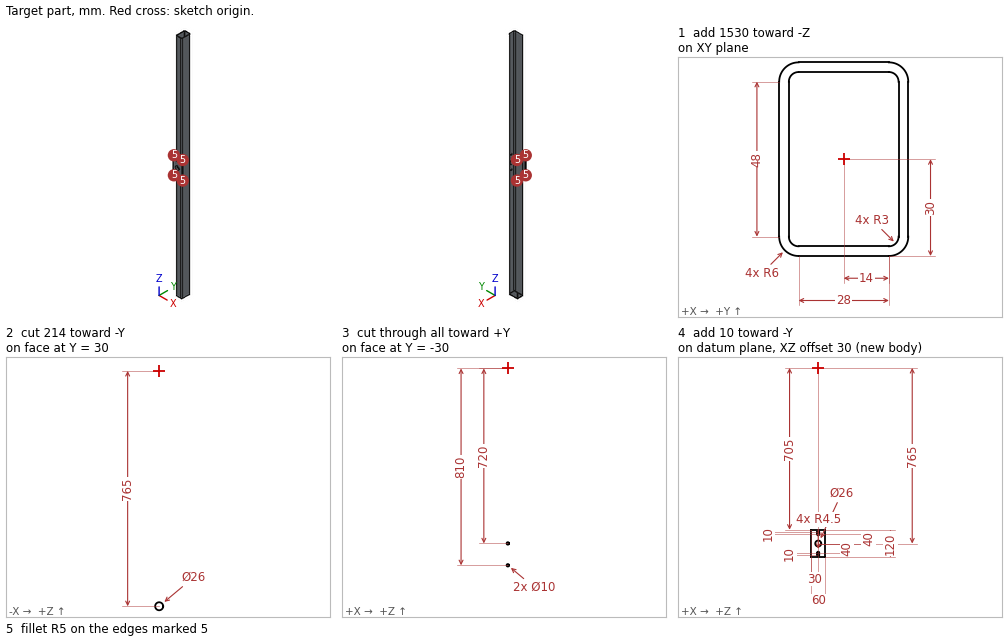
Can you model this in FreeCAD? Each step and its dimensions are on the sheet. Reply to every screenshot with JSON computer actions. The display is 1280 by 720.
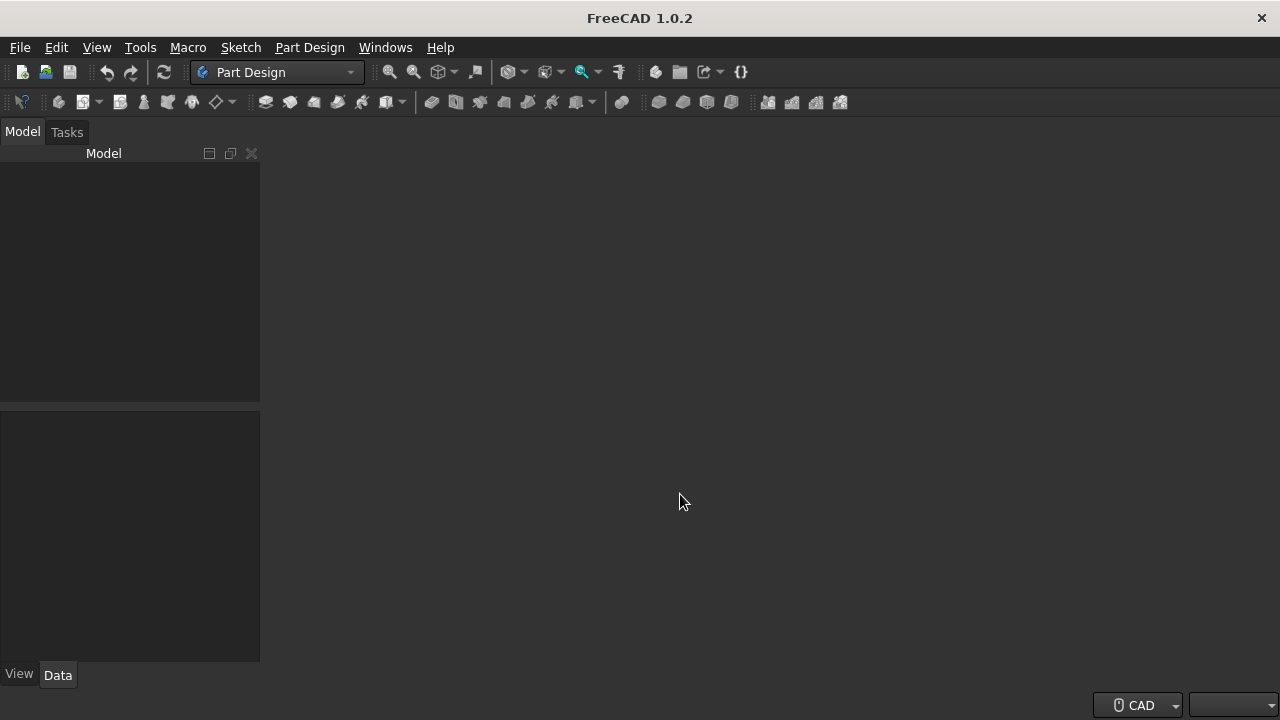
{"action": "left_click", "coordinate": [22, 72]}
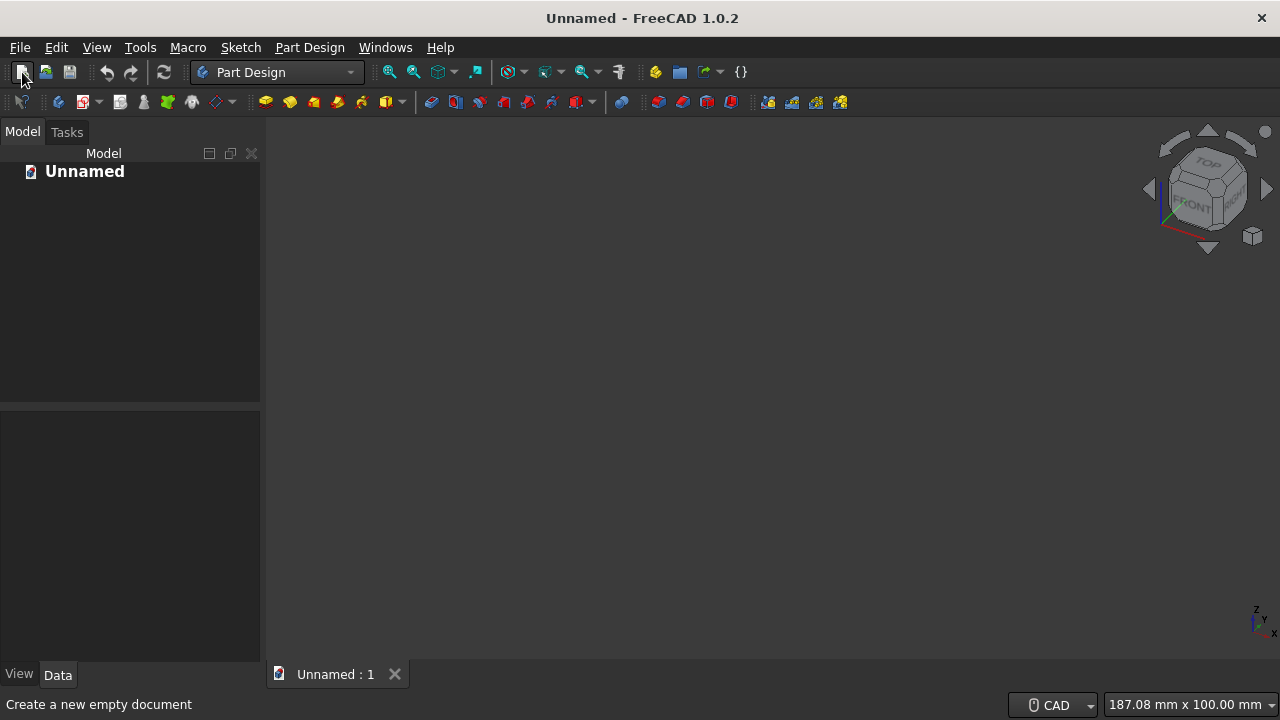
{"action": "left_click", "coordinate": [84, 102]}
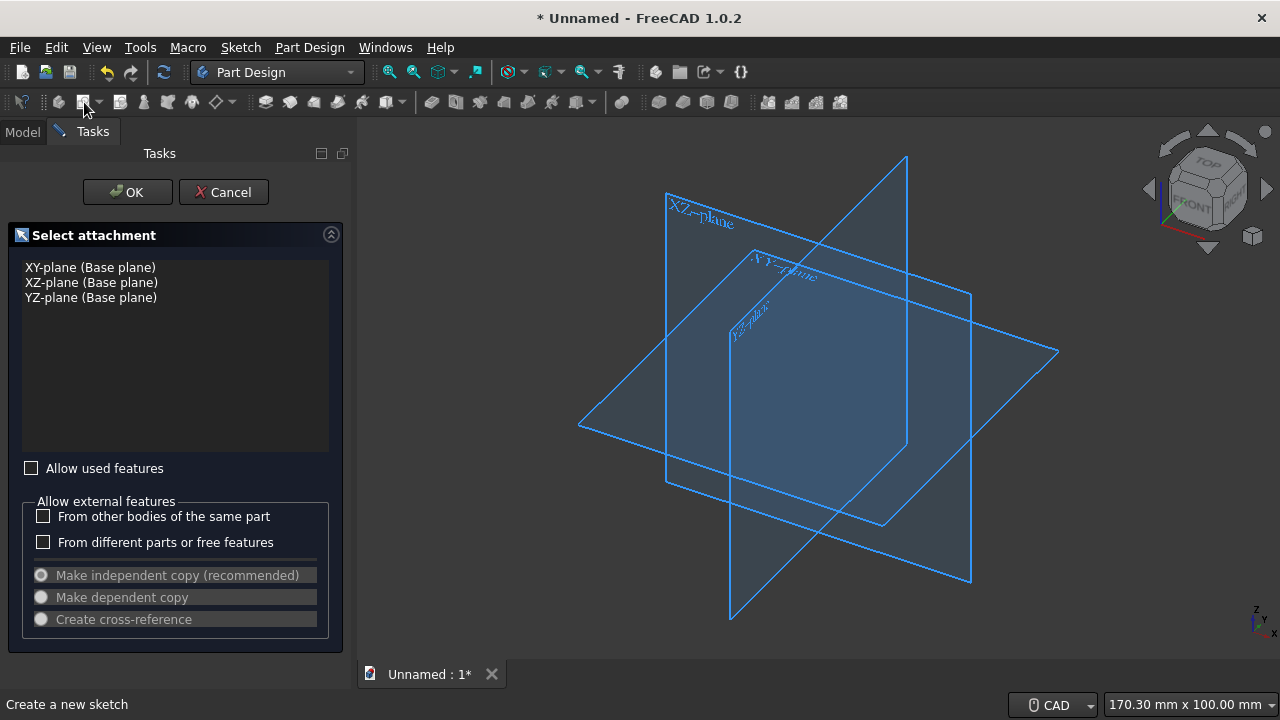
{"action": "left_click", "coordinate": [82, 268]}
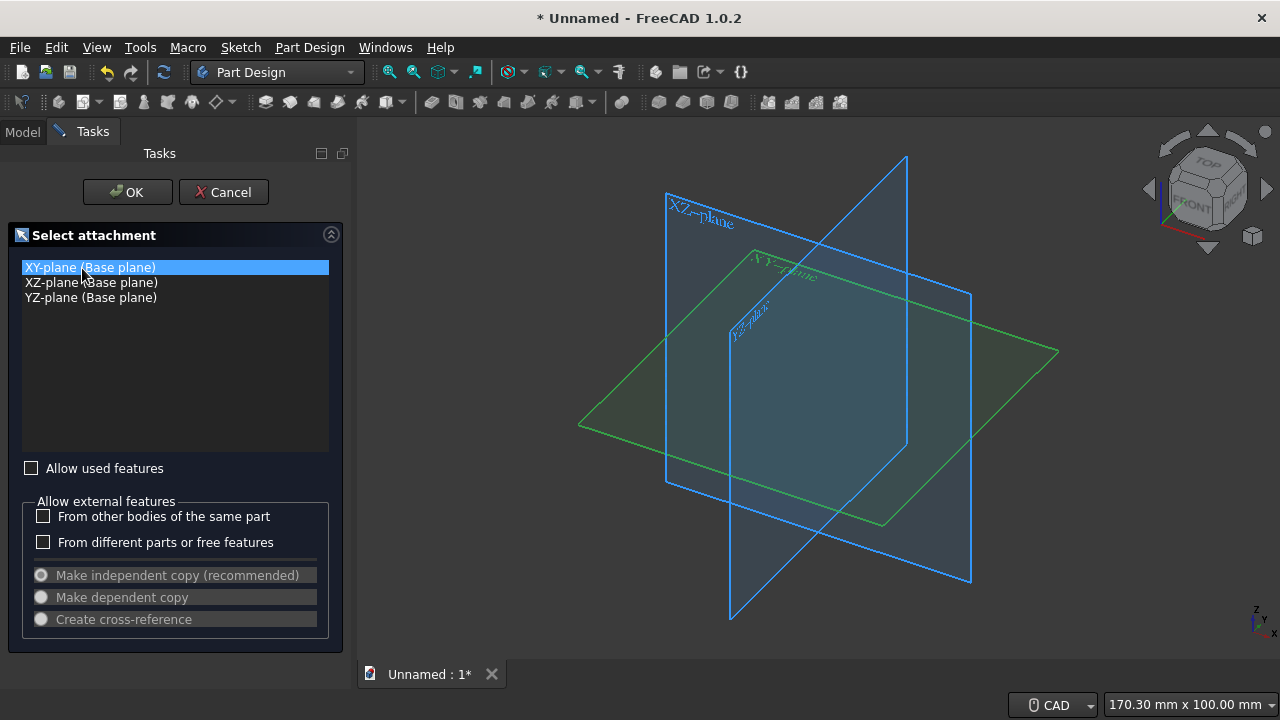
{"action": "left_click", "coordinate": [128, 192]}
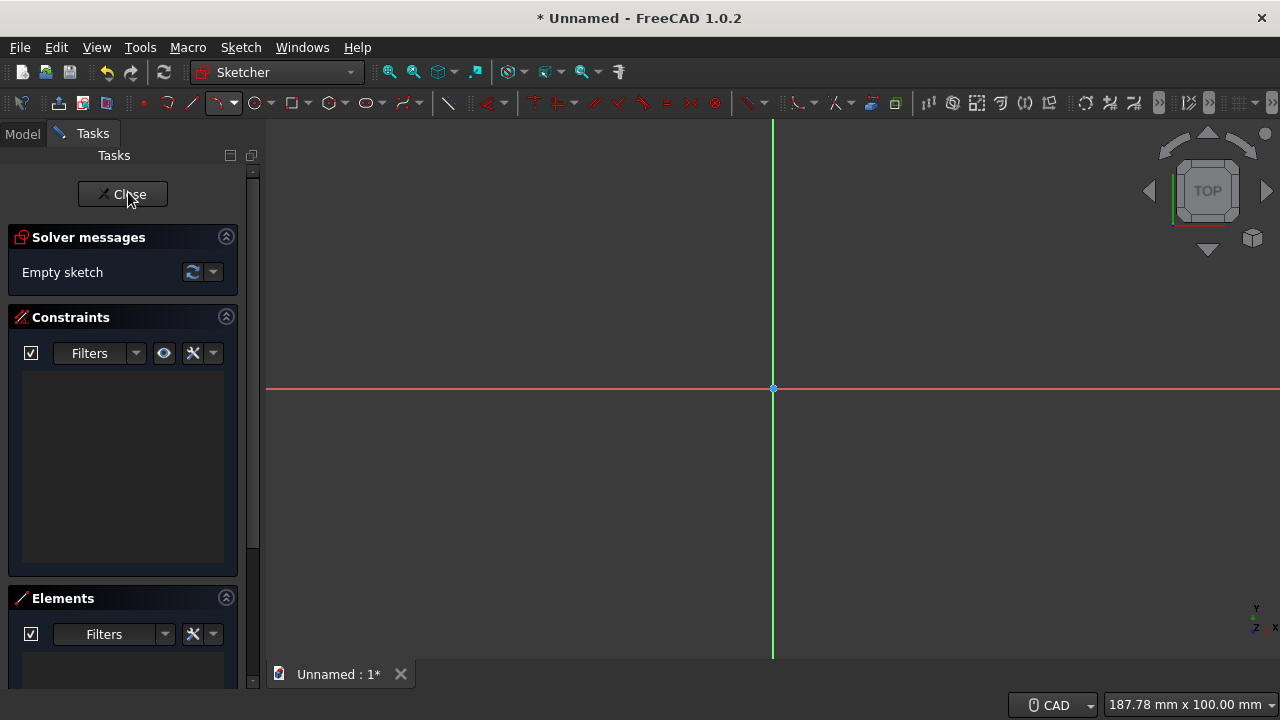
{"action": "left_click", "coordinate": [192, 104]}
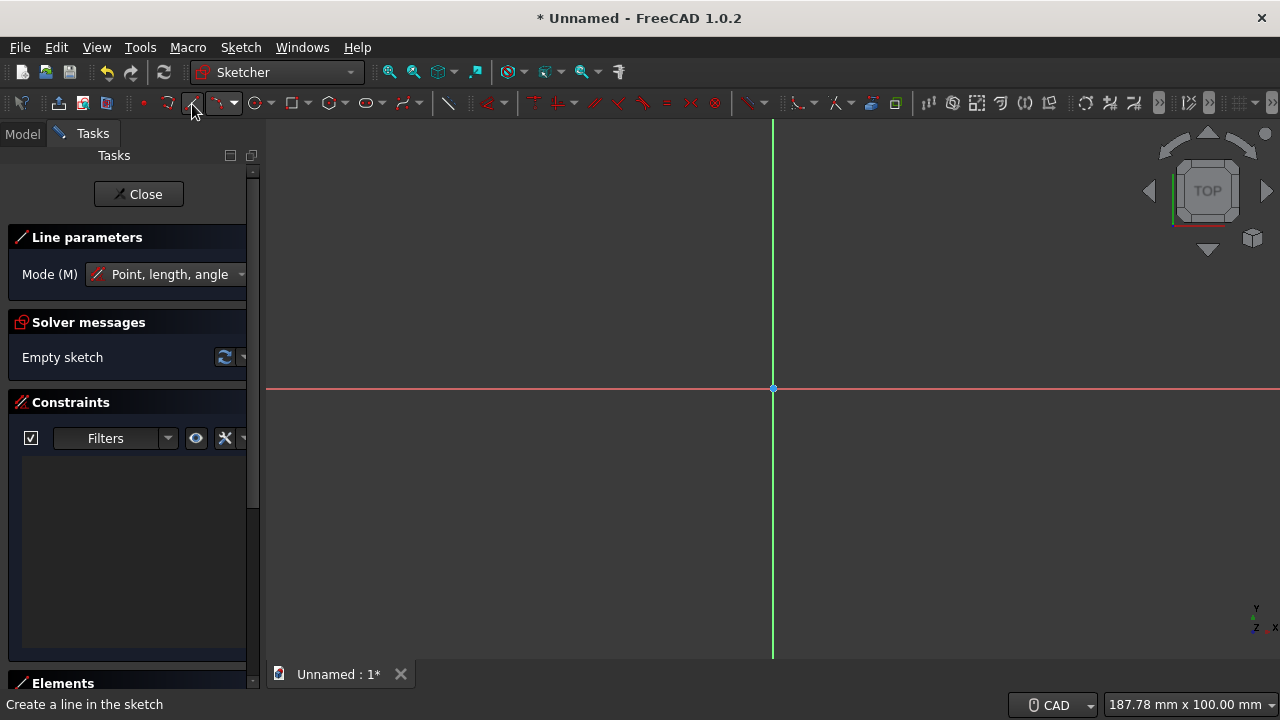
{"action": "left_click", "coordinate": [849, 551]}
{"action": "left_click", "coordinate": [697, 551]}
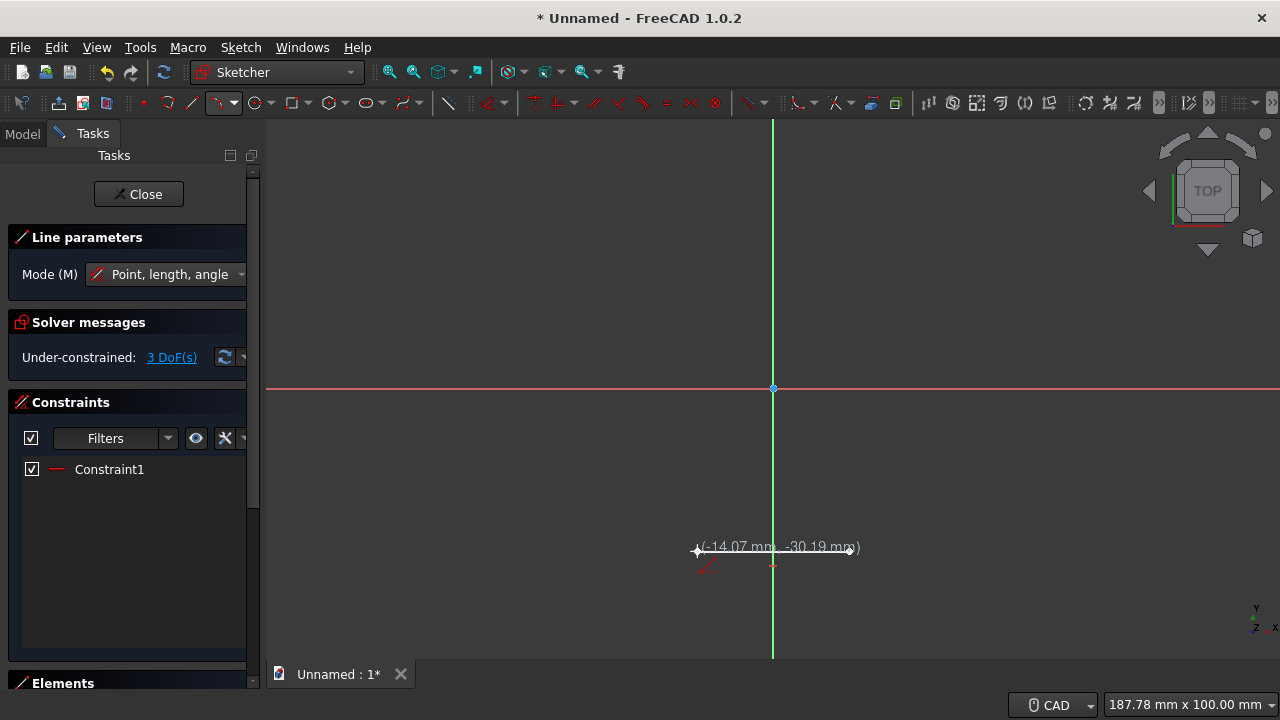
{"action": "left_click", "coordinate": [665, 519]}
{"action": "left_click", "coordinate": [665, 259]}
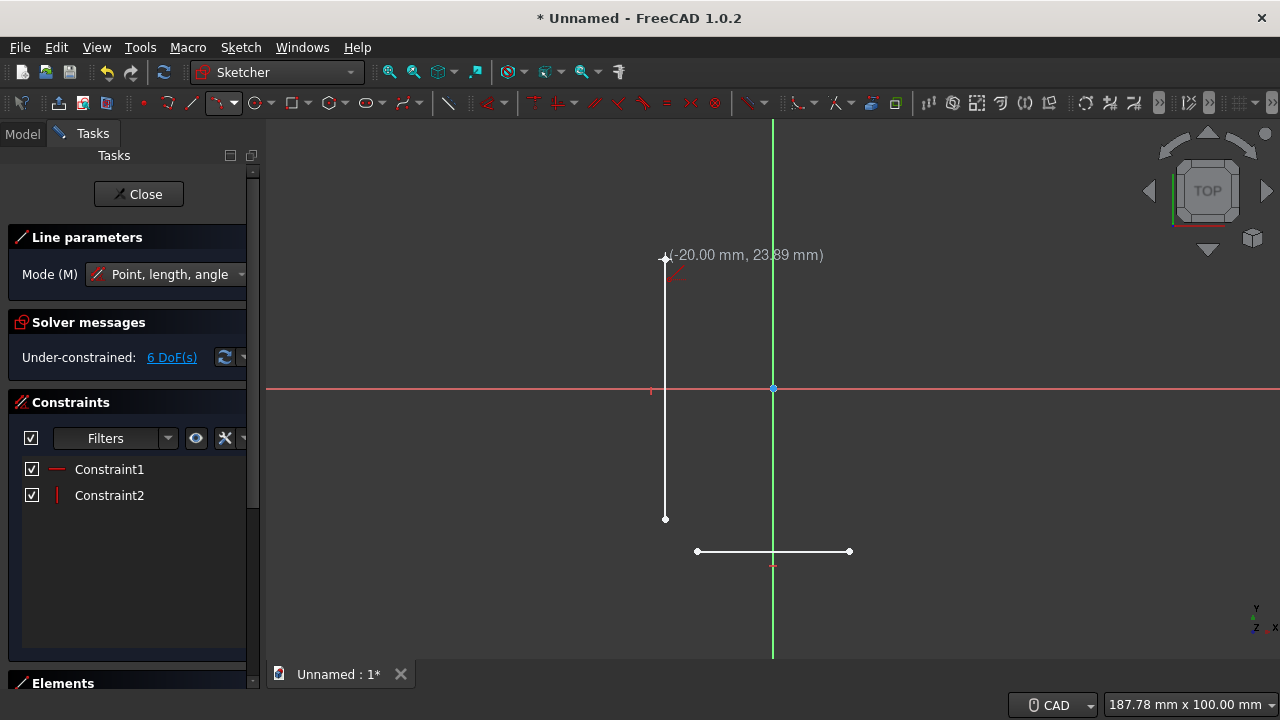
{"action": "left_click", "coordinate": [697, 227]}
{"action": "left_click", "coordinate": [849, 227]}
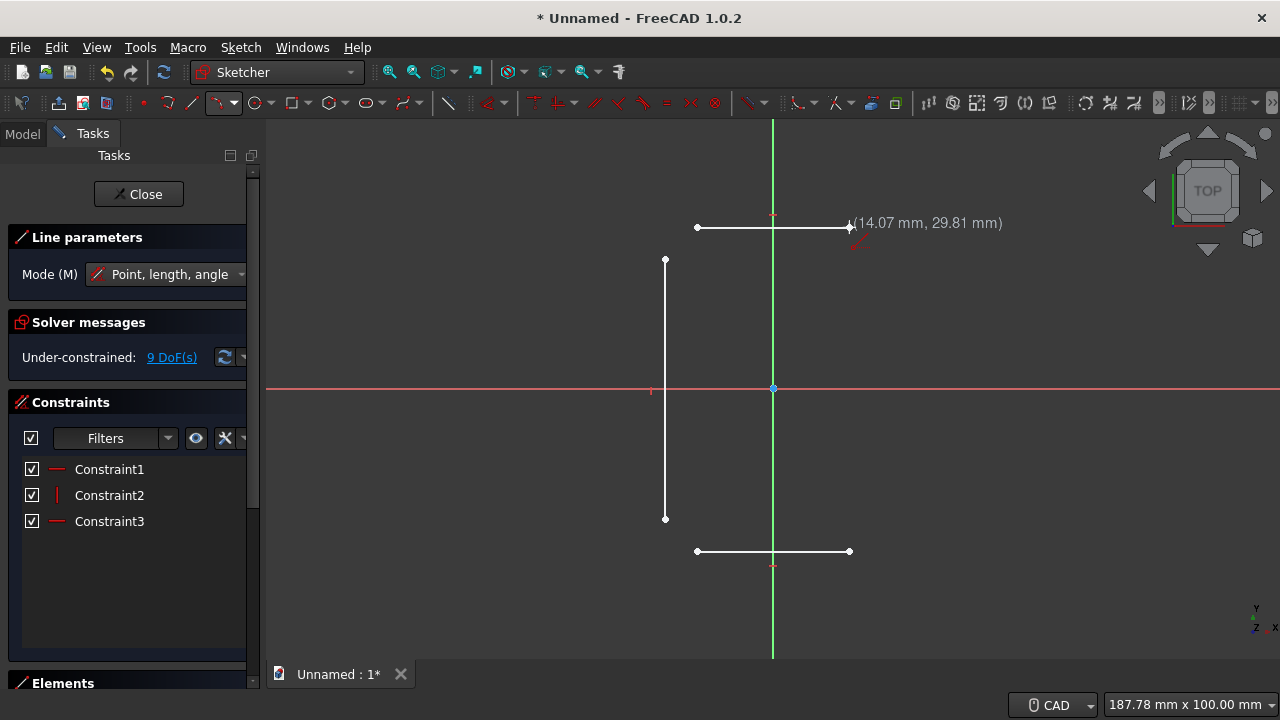
{"action": "left_click", "coordinate": [881, 259]}
{"action": "left_click", "coordinate": [881, 519]}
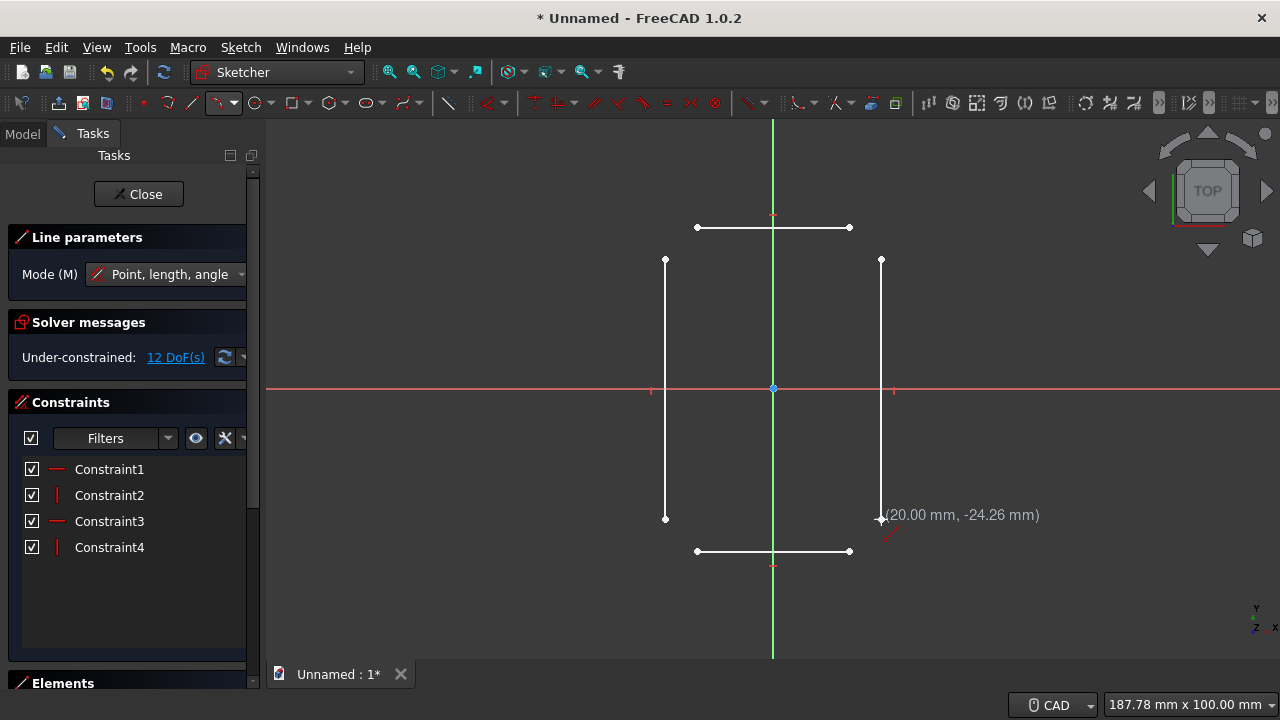
{"action": "left_click", "coordinate": [218, 104]}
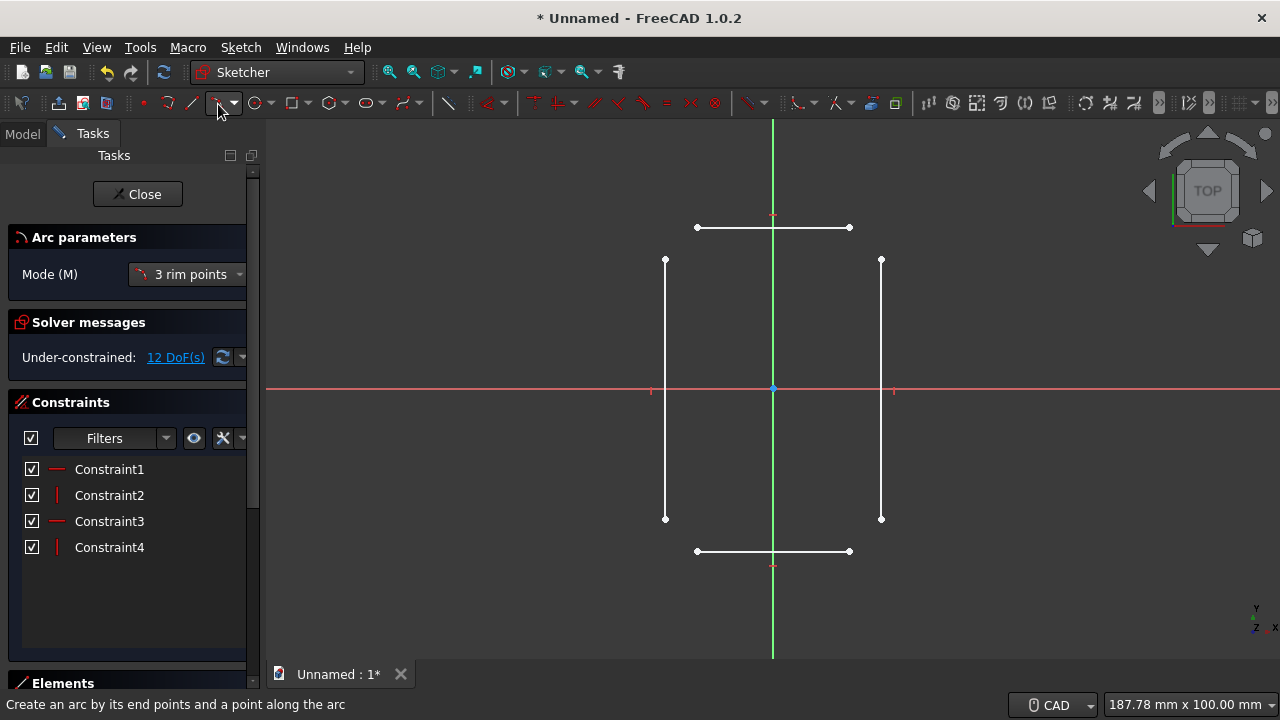
{"action": "left_click", "coordinate": [697, 552]}
{"action": "left_click", "coordinate": [665, 520]}